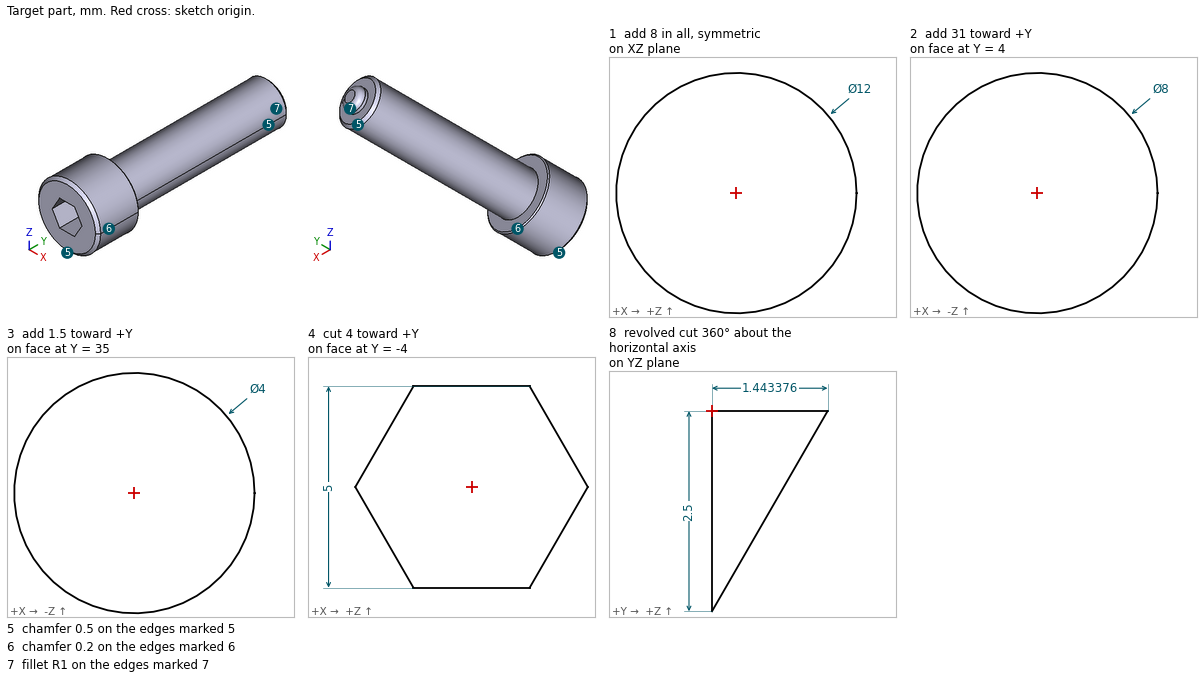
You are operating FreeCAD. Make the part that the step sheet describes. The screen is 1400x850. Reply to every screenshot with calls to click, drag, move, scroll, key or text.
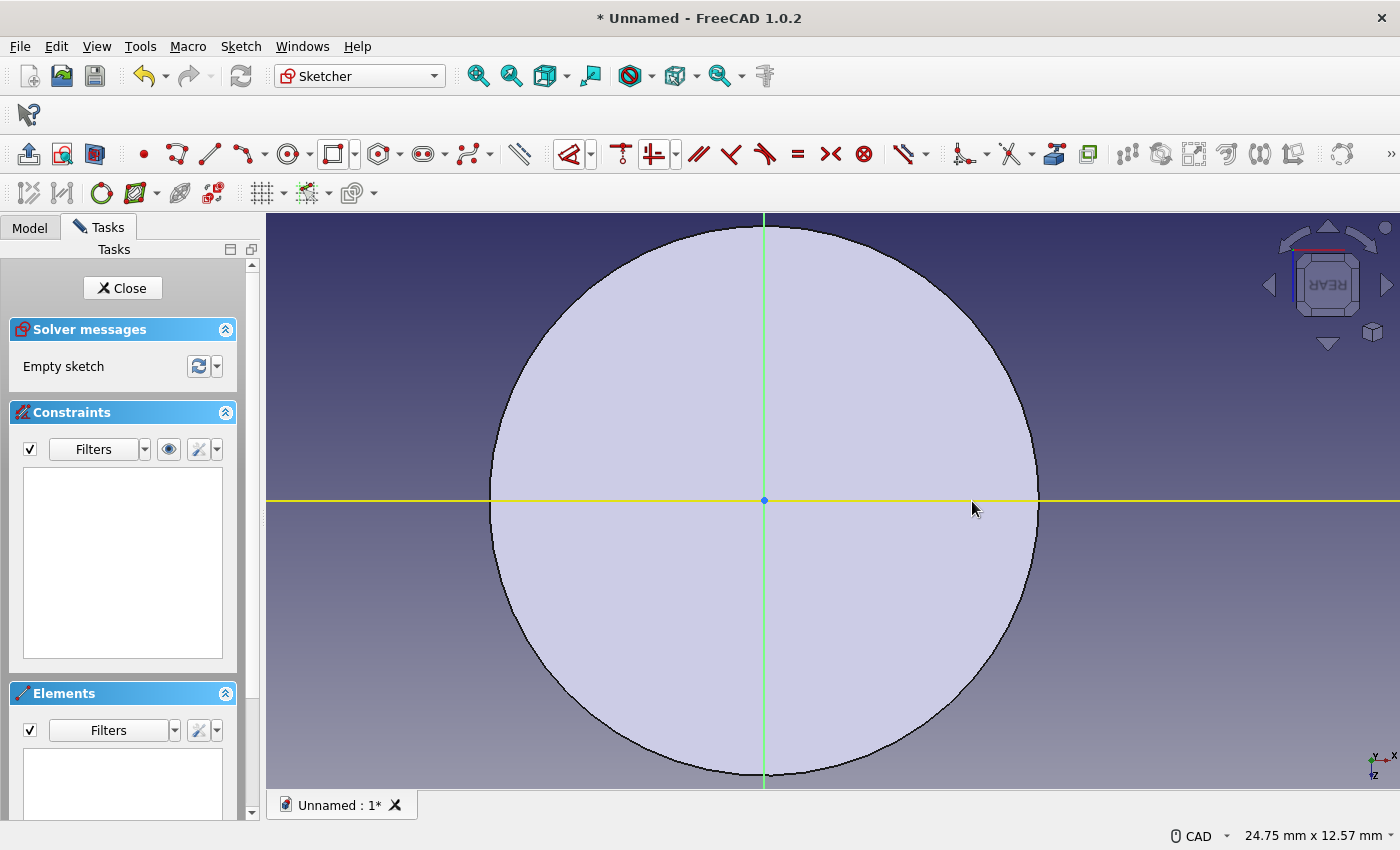
click(288, 154)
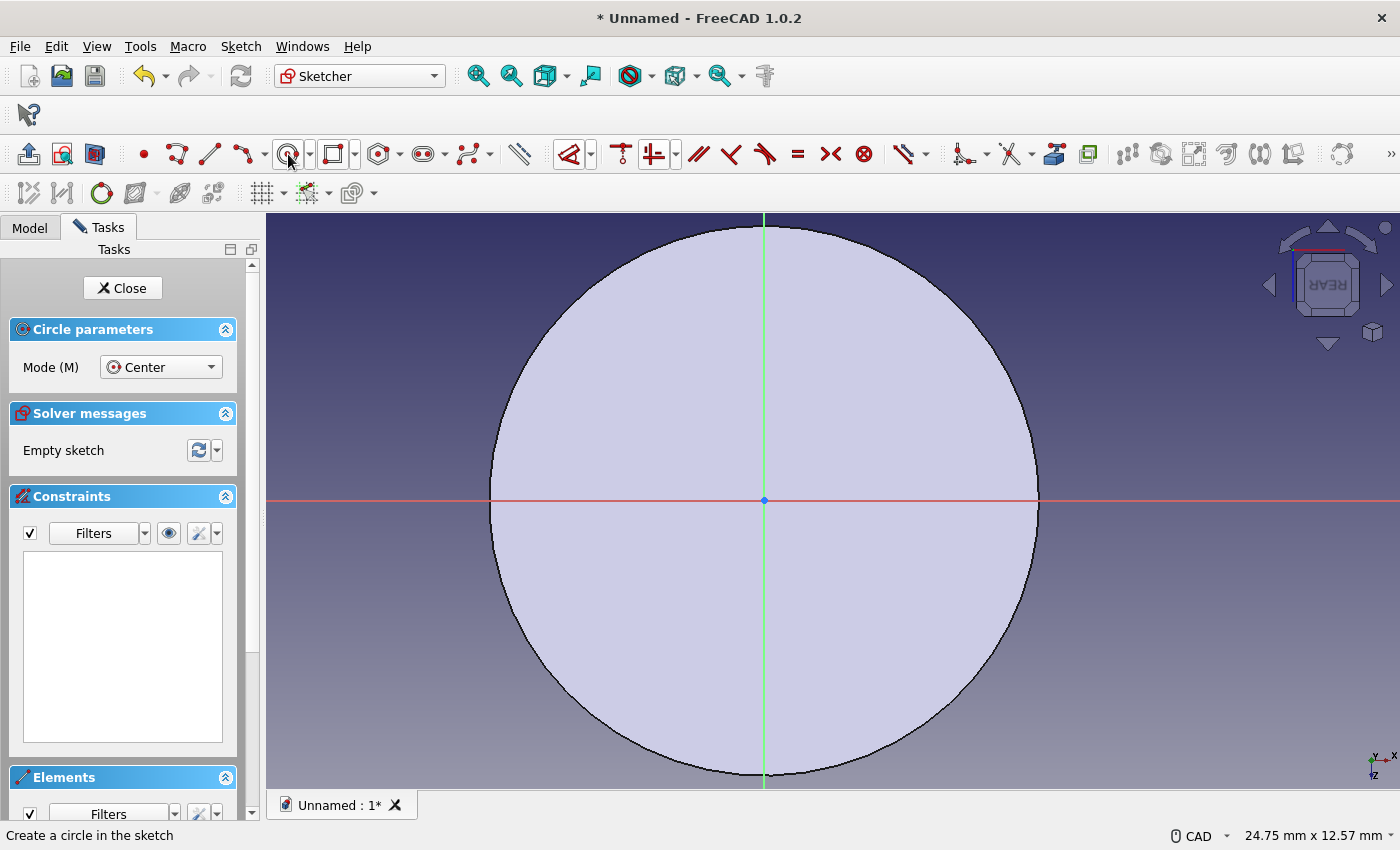
click(764, 501)
move(894, 371)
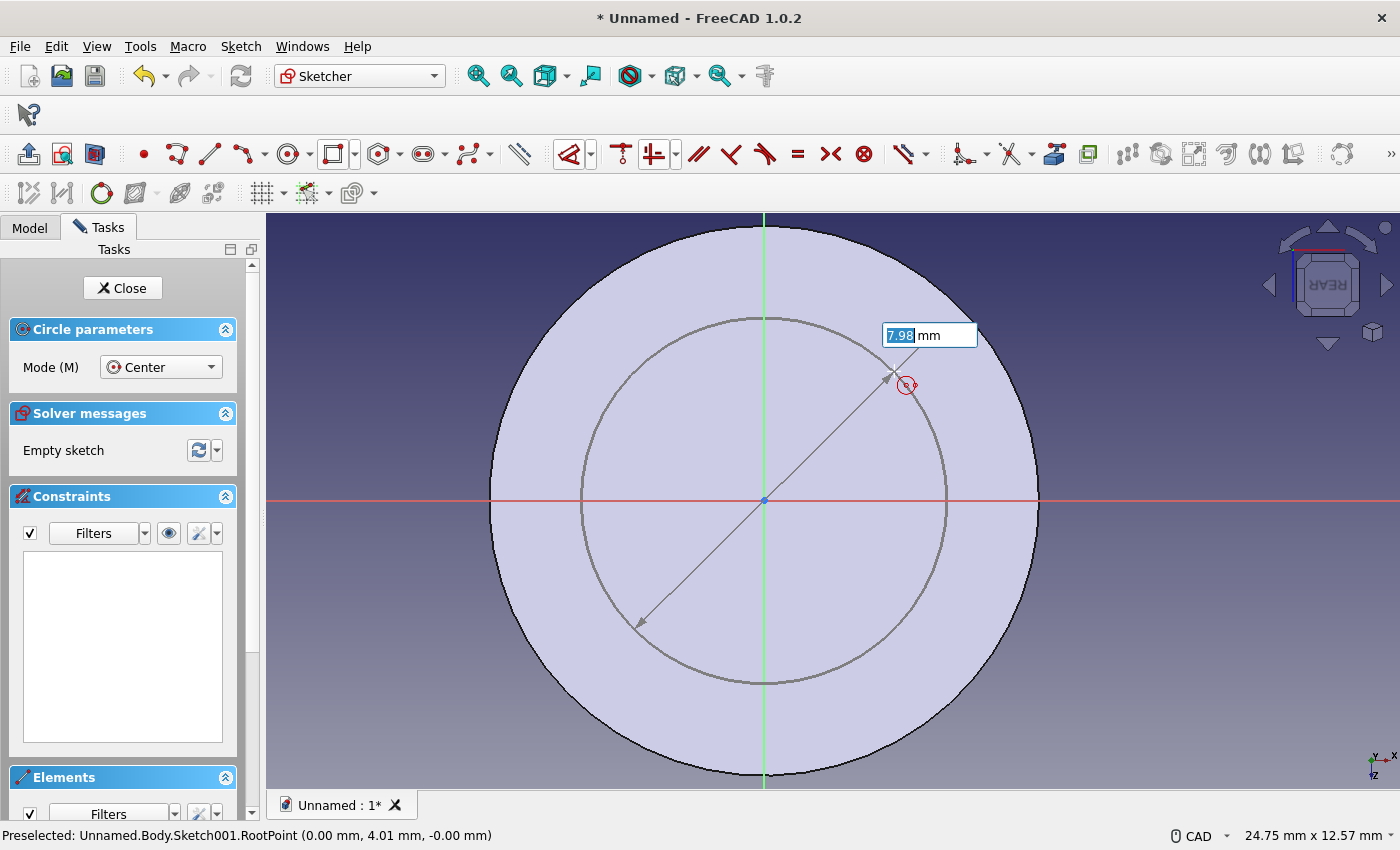
text(8)
key(Return)
key(Escape)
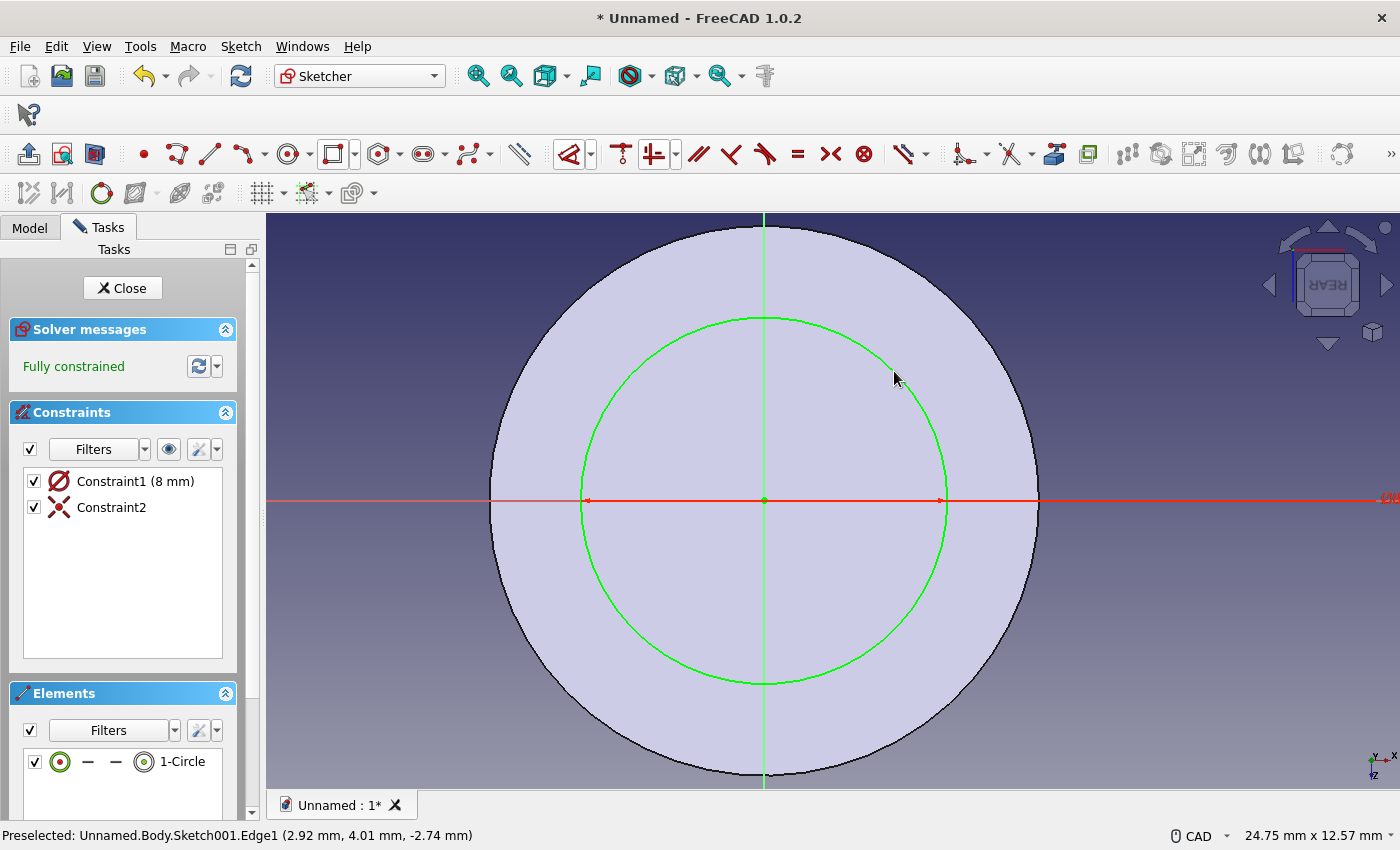
click(123, 288)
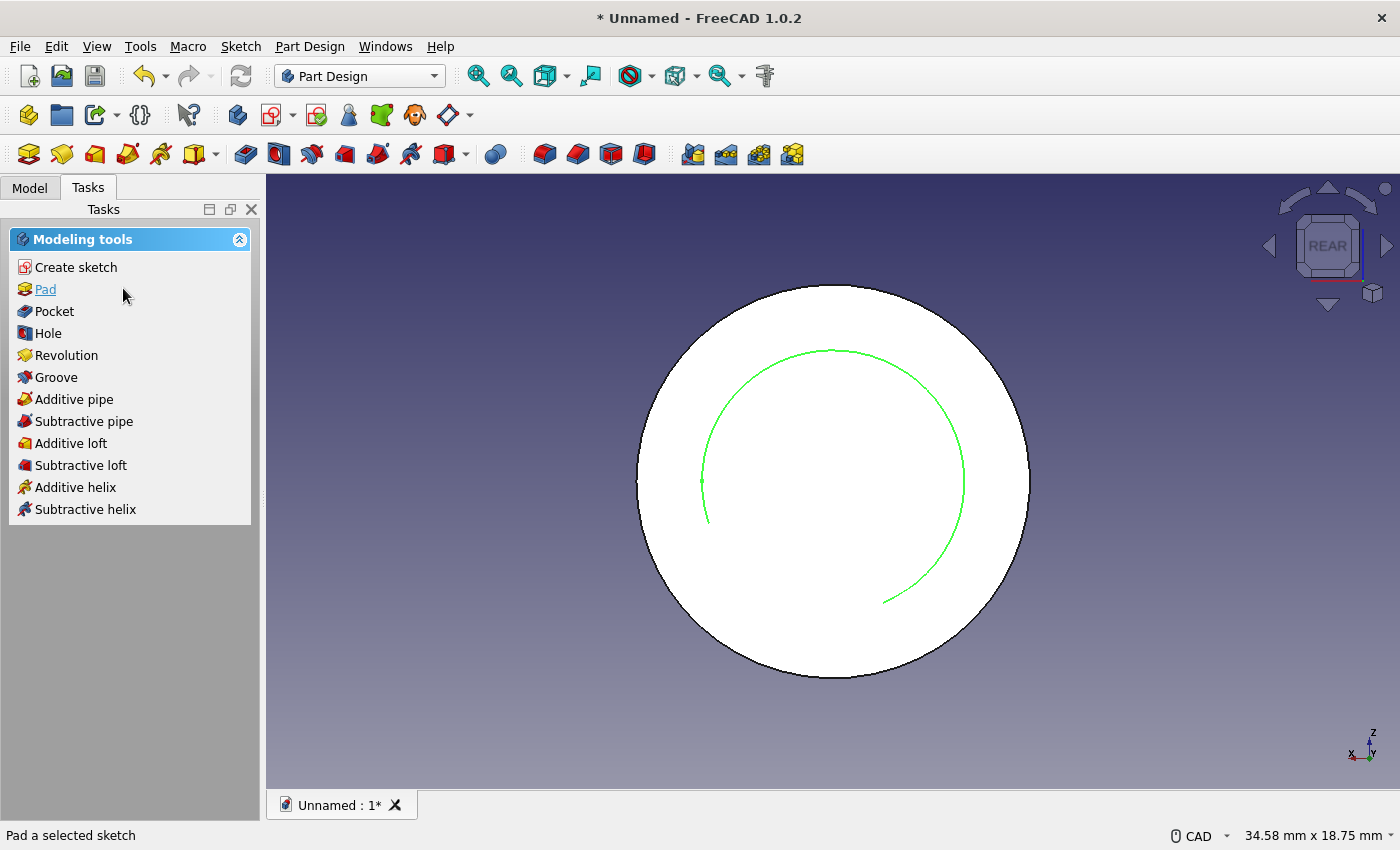
click(29, 154)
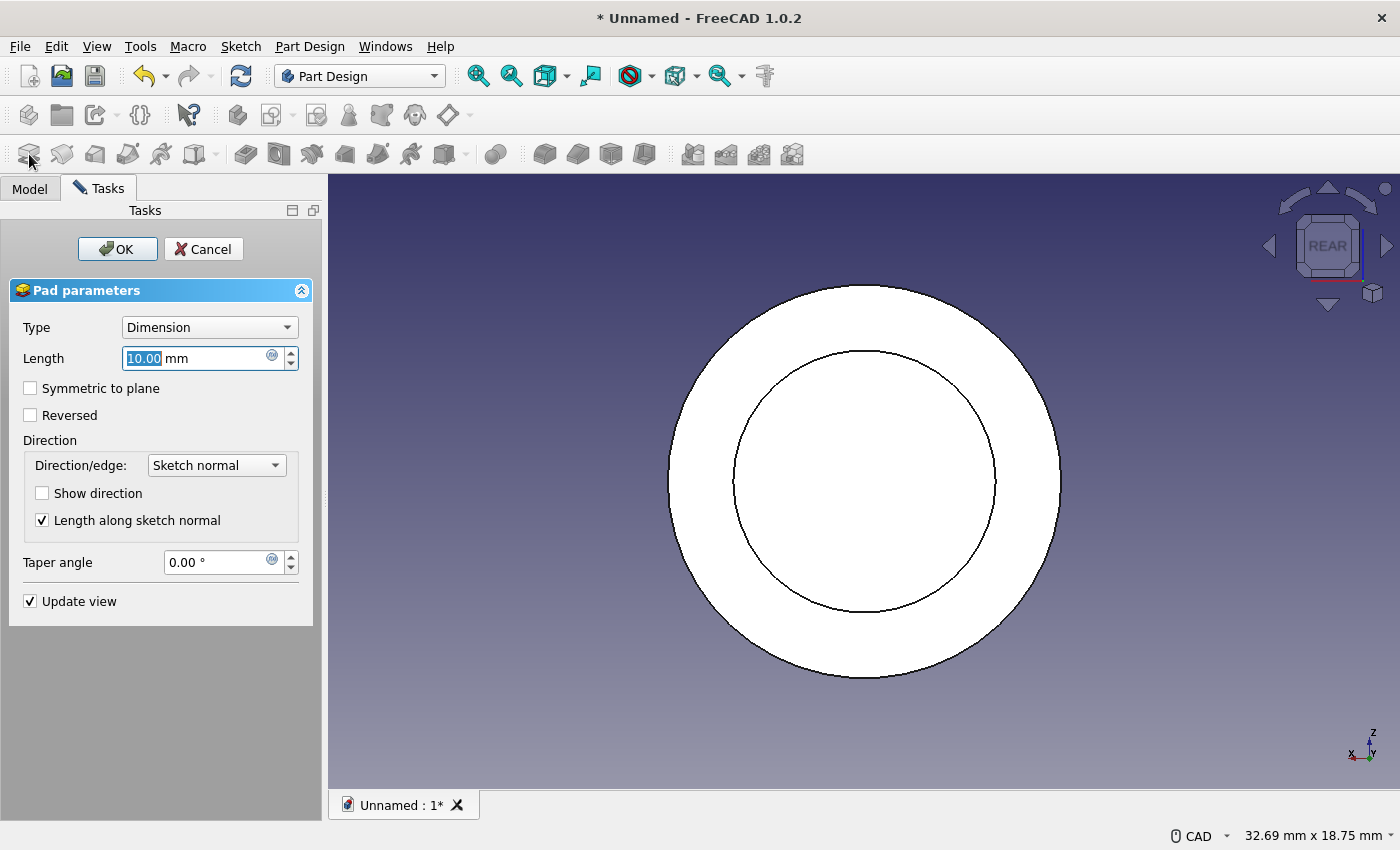
text(31)
key(Tab)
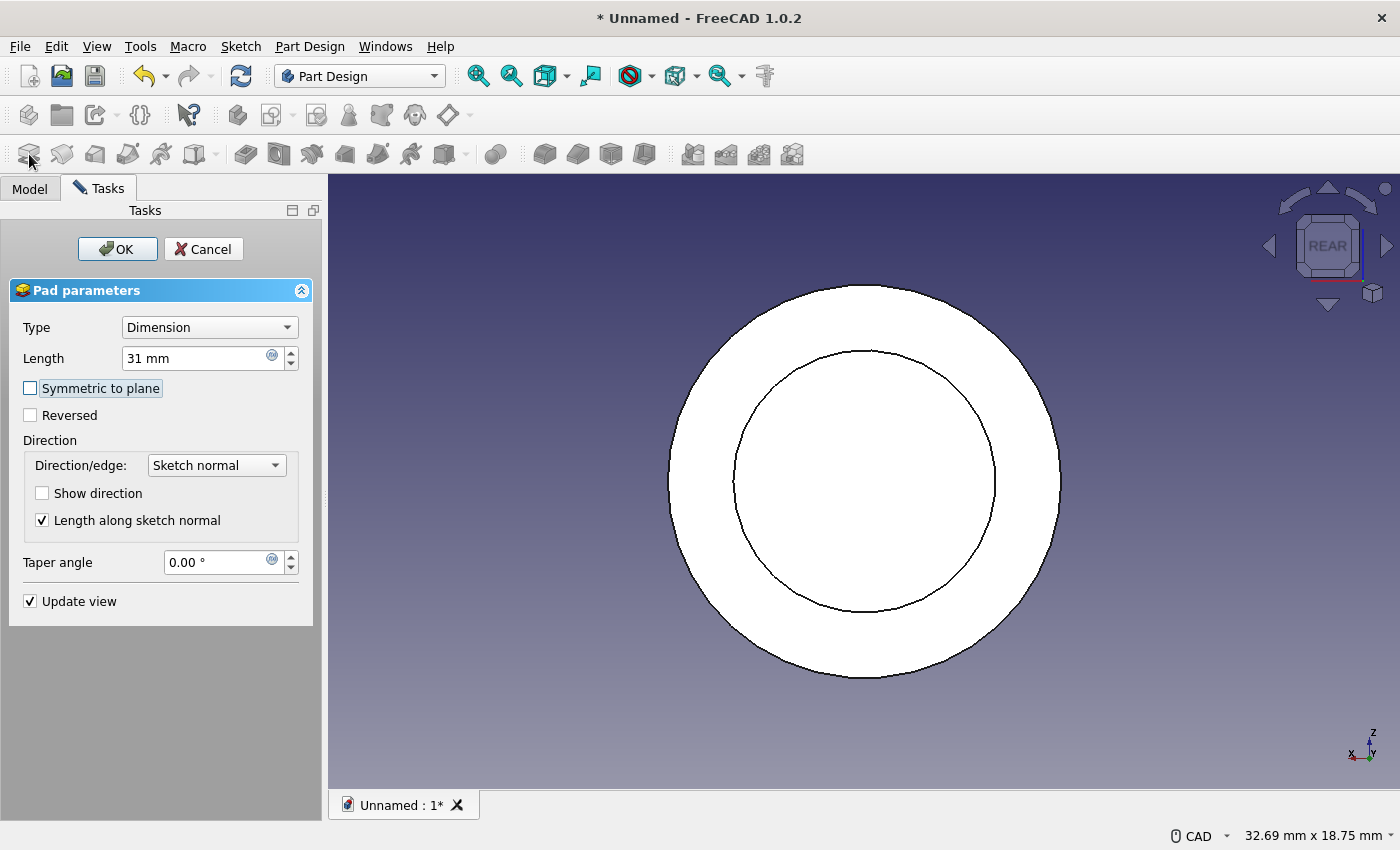
click(118, 249)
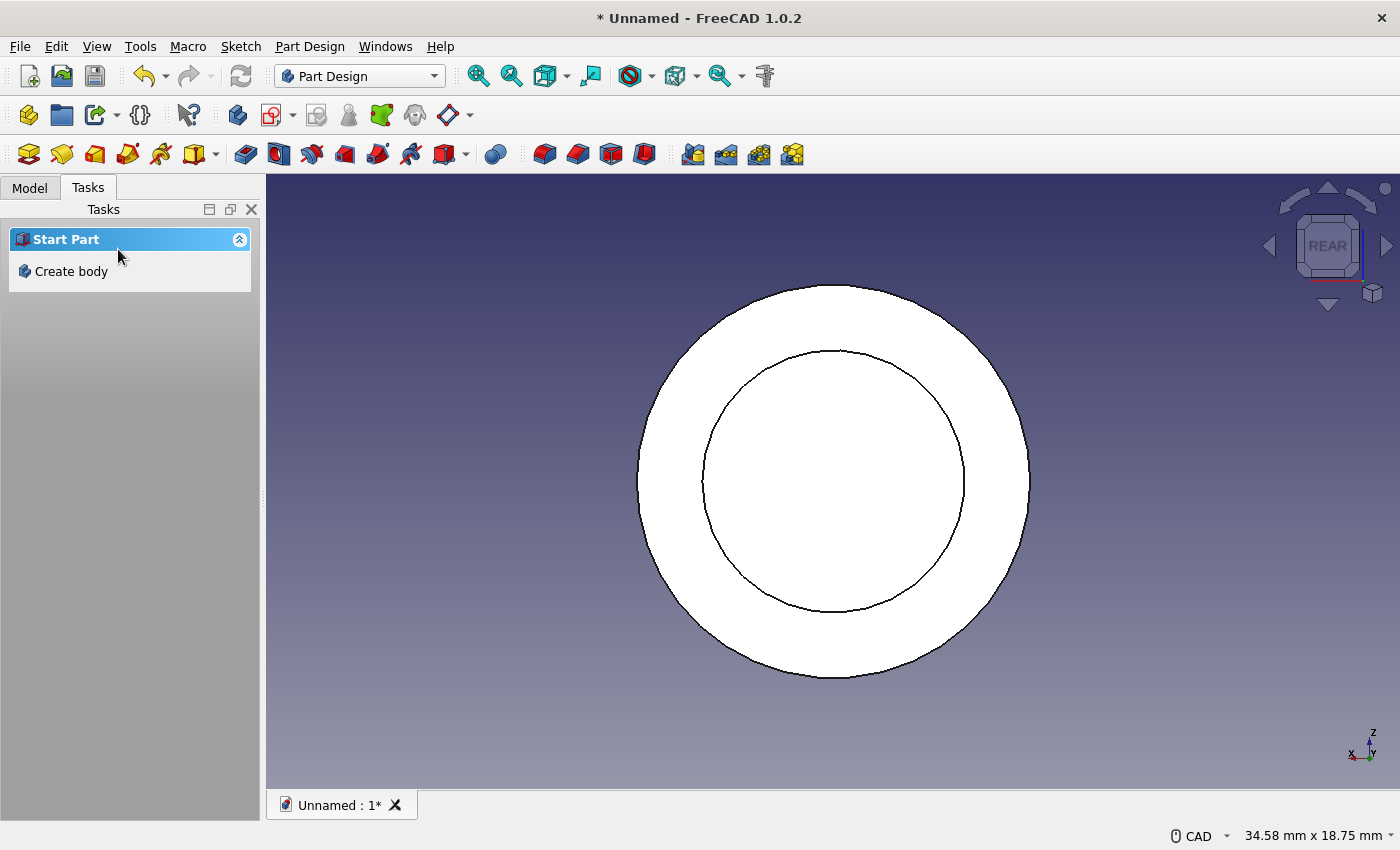
click(833, 481)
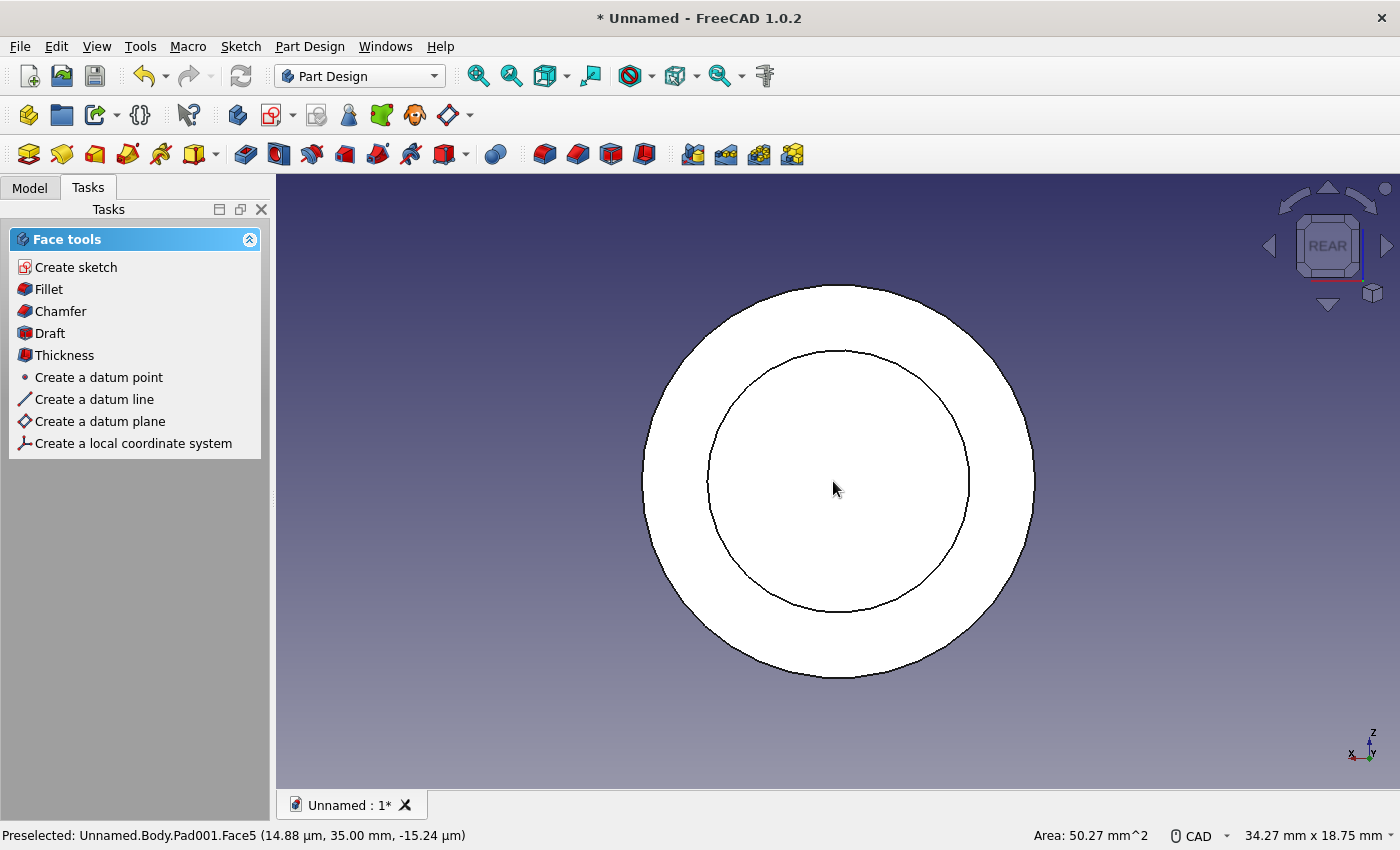
click(270, 116)